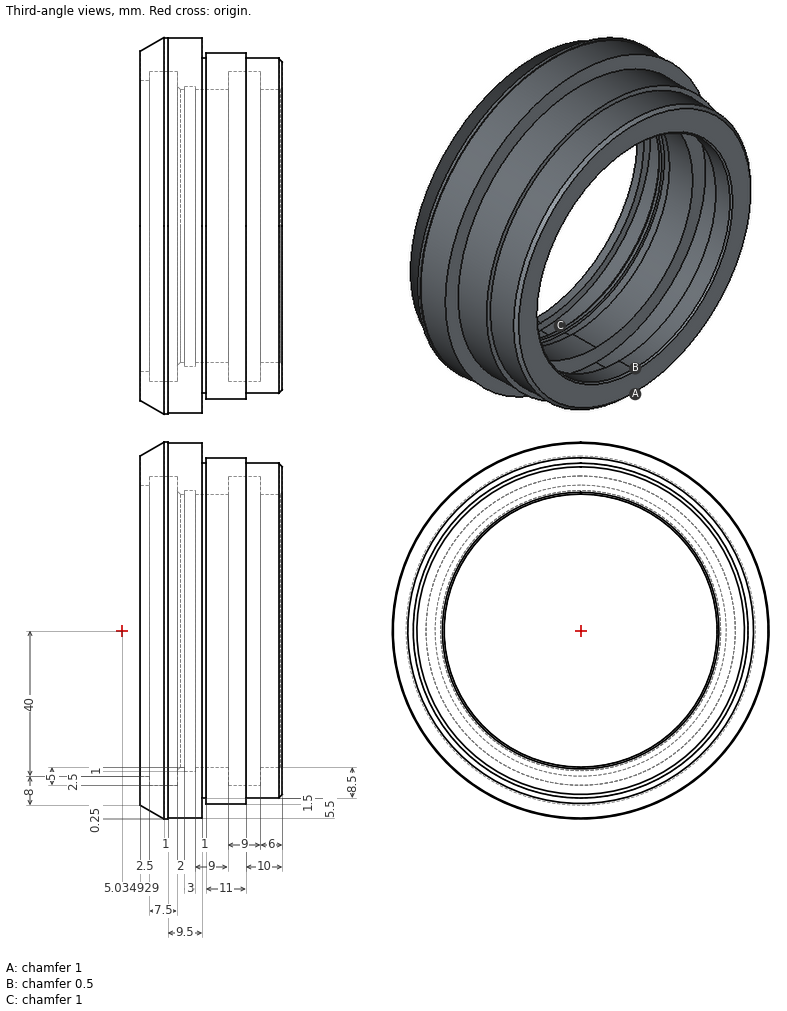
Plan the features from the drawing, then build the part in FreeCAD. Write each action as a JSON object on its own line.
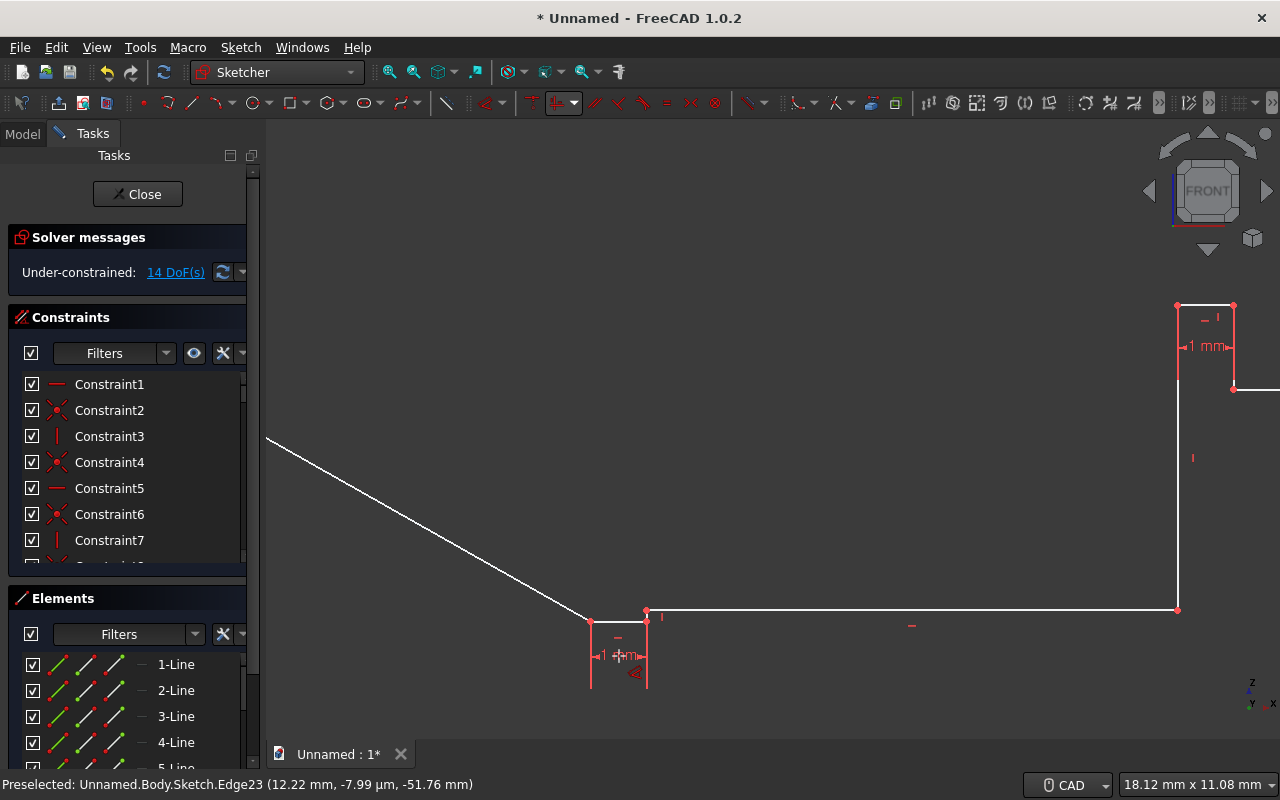
{"action": "scroll", "coordinate": [630, 626], "scroll_direction": "down", "scroll_amount": 10}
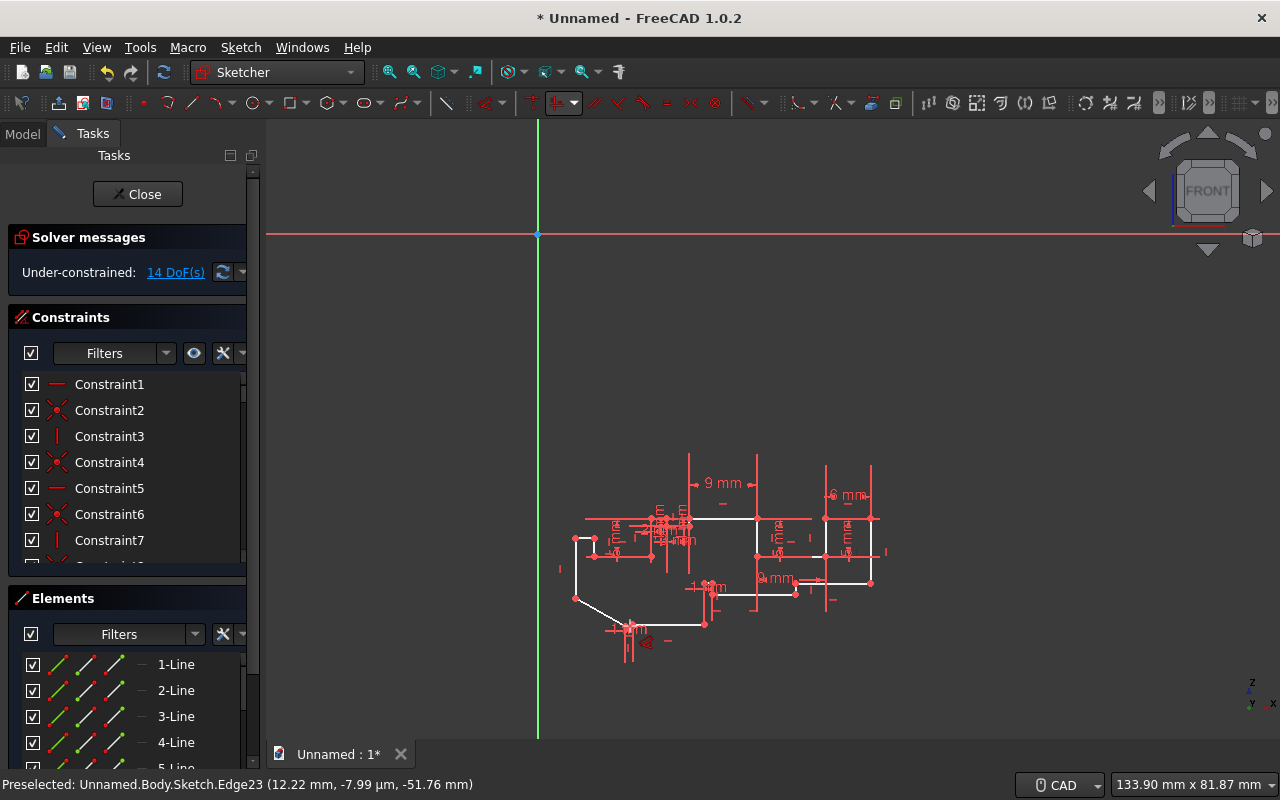
{"action": "left_click", "coordinate": [576, 580]}
{"action": "left_click", "coordinate": [610, 582]}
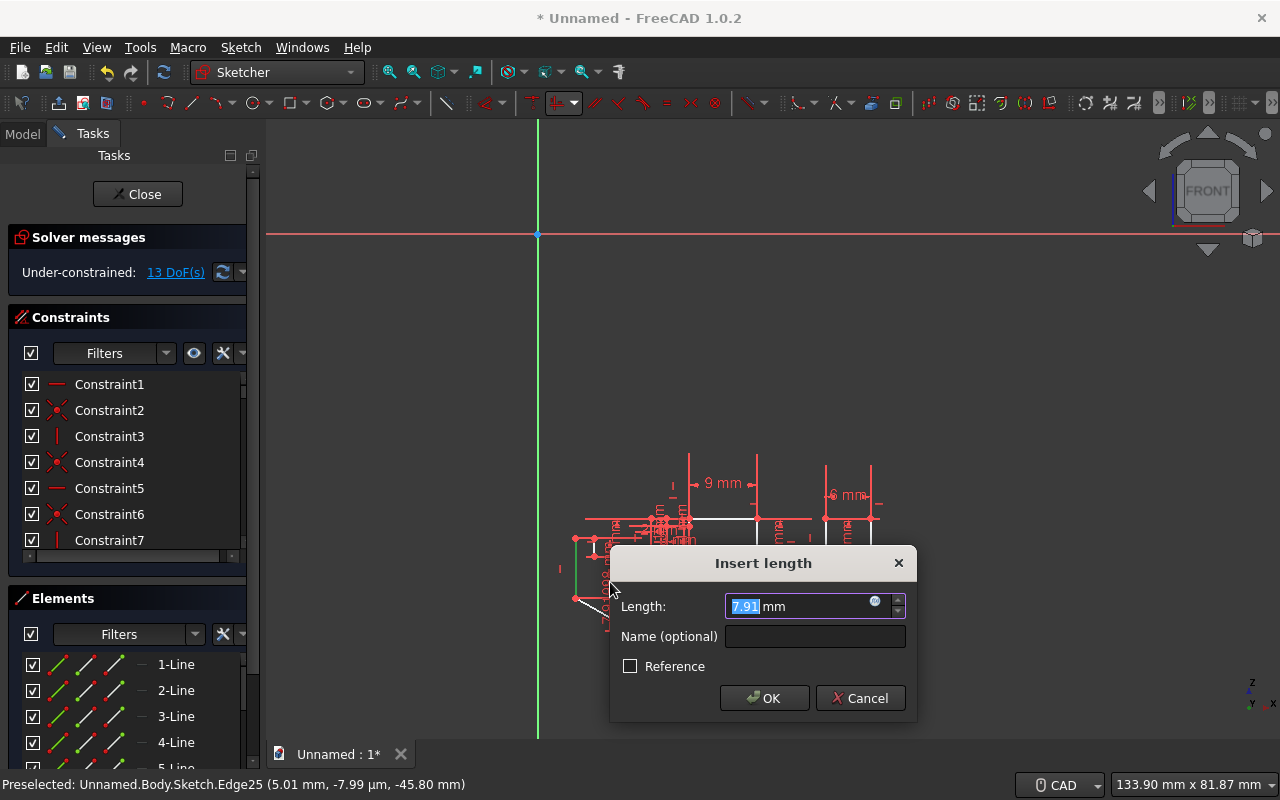
{"action": "type", "text": "8"}
{"action": "key", "text": "Return"}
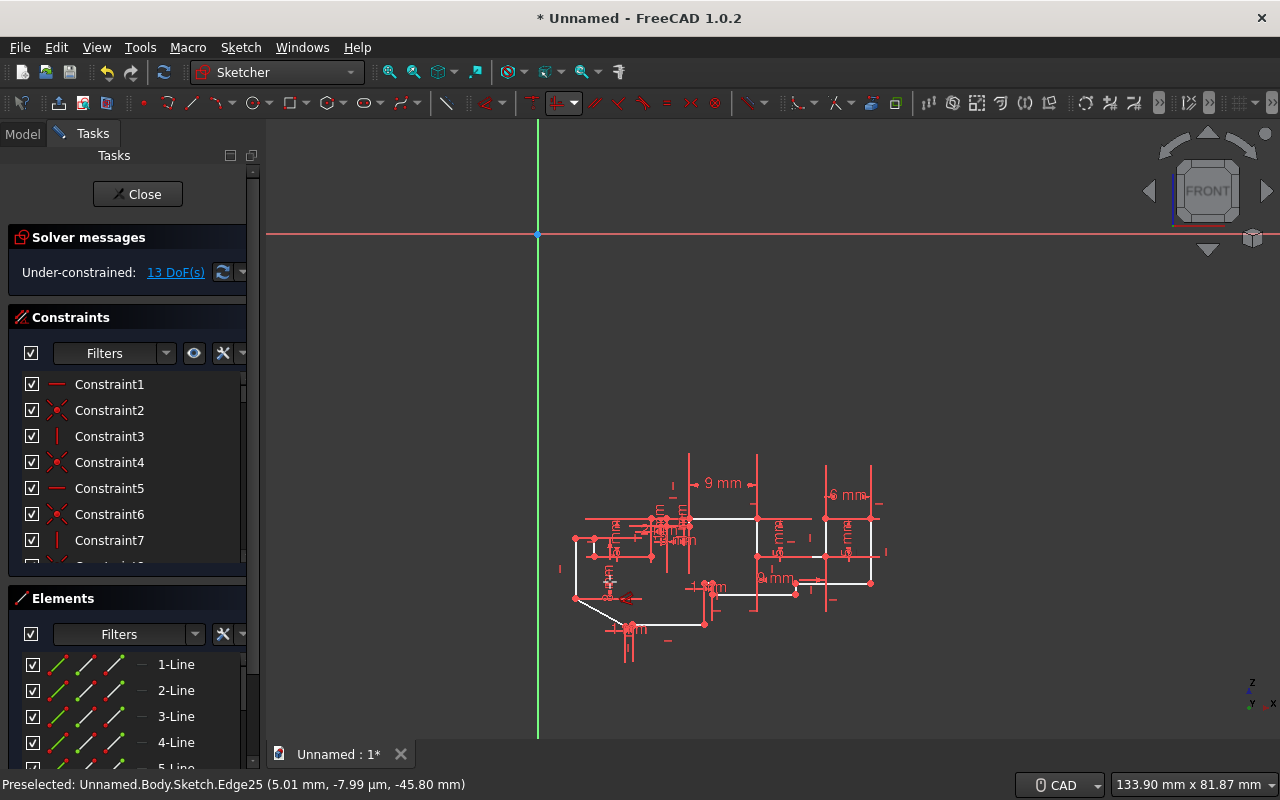
{"action": "left_click", "coordinate": [848, 584]}
{"action": "left_click", "coordinate": [833, 618]}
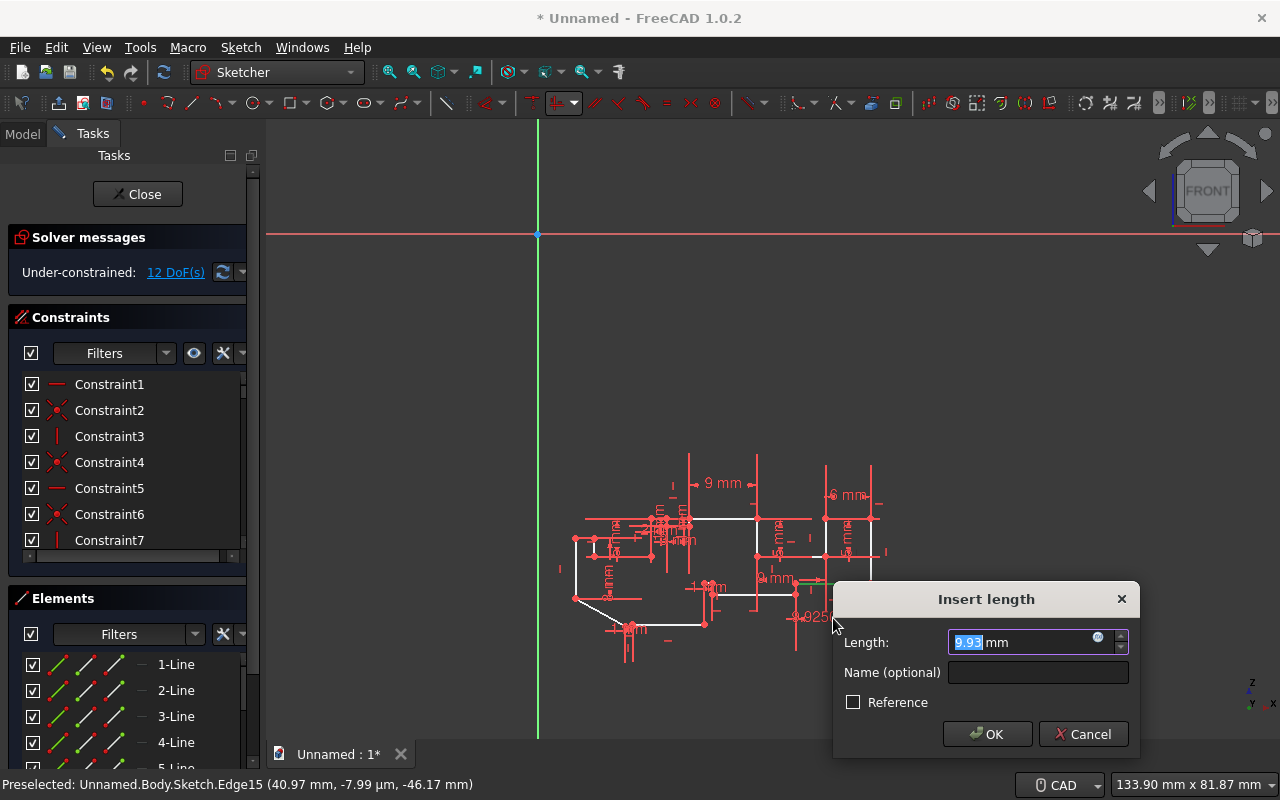
{"action": "type", "text": "10"}
{"action": "key", "text": "Return"}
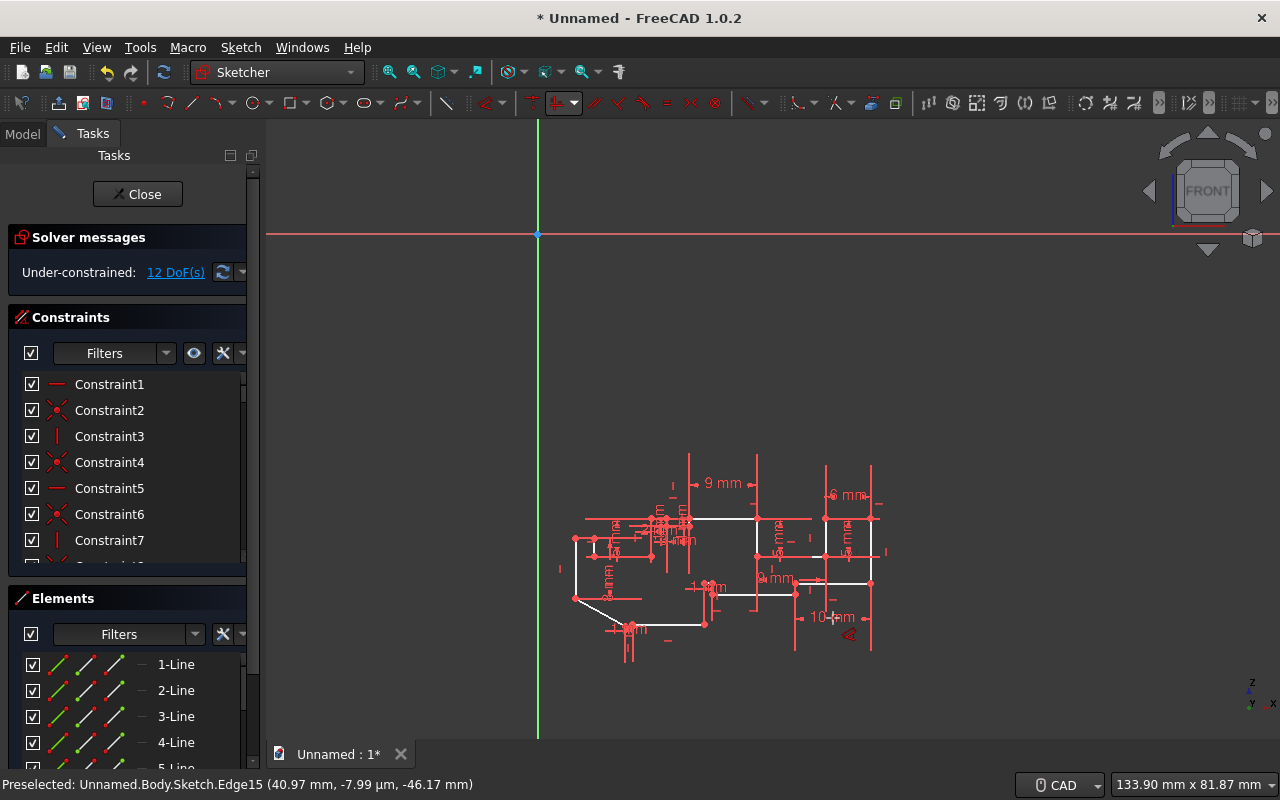
{"action": "left_click", "coordinate": [770, 595]}
{"action": "left_click", "coordinate": [754, 629]}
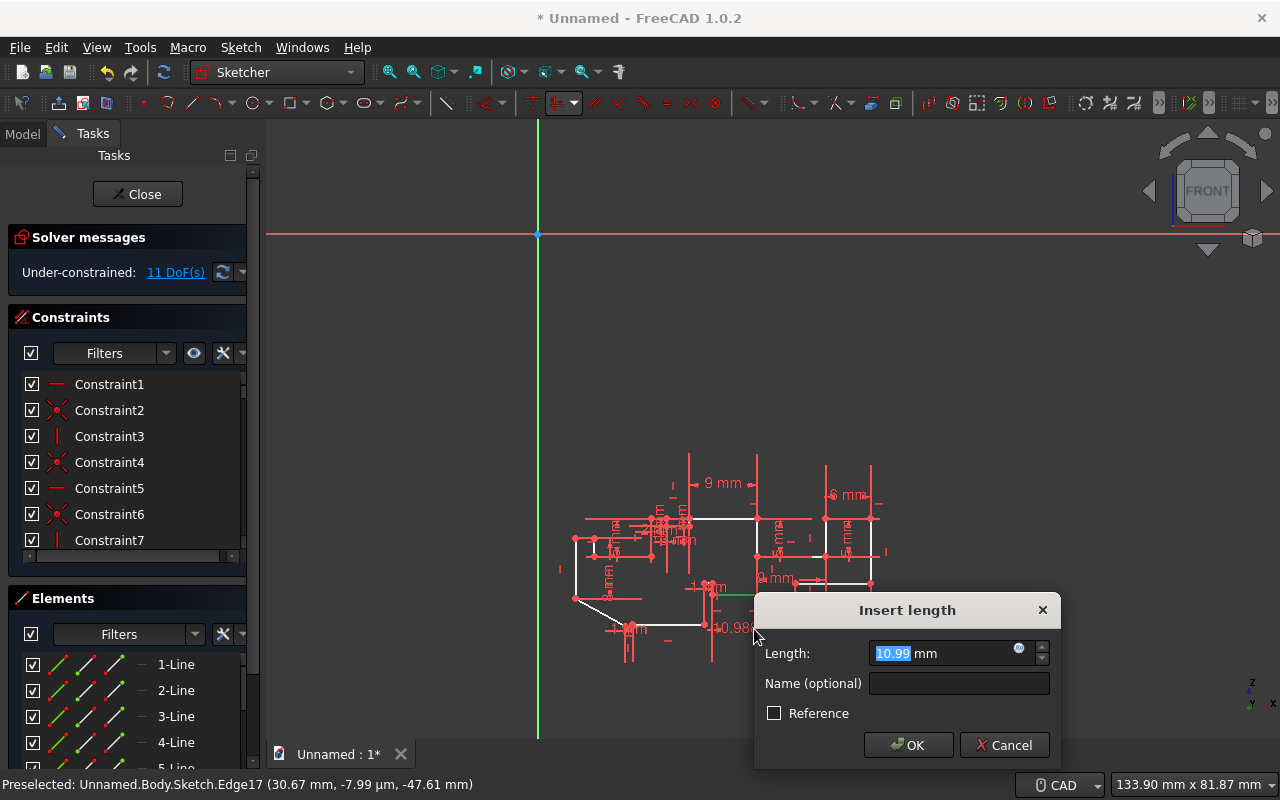
{"action": "type", "text": "11"}
{"action": "key", "text": "Return"}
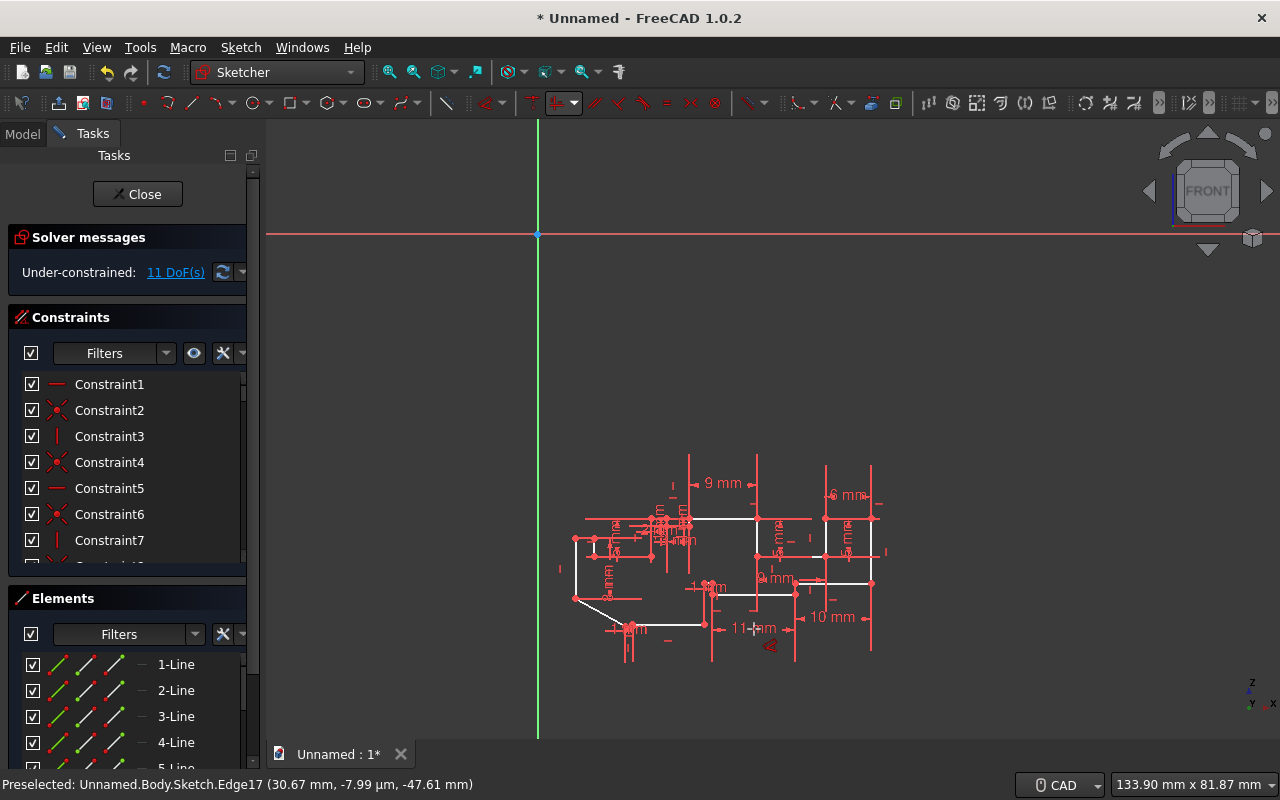
{"action": "scroll", "coordinate": [585, 538], "scroll_direction": "up", "scroll_amount": 4}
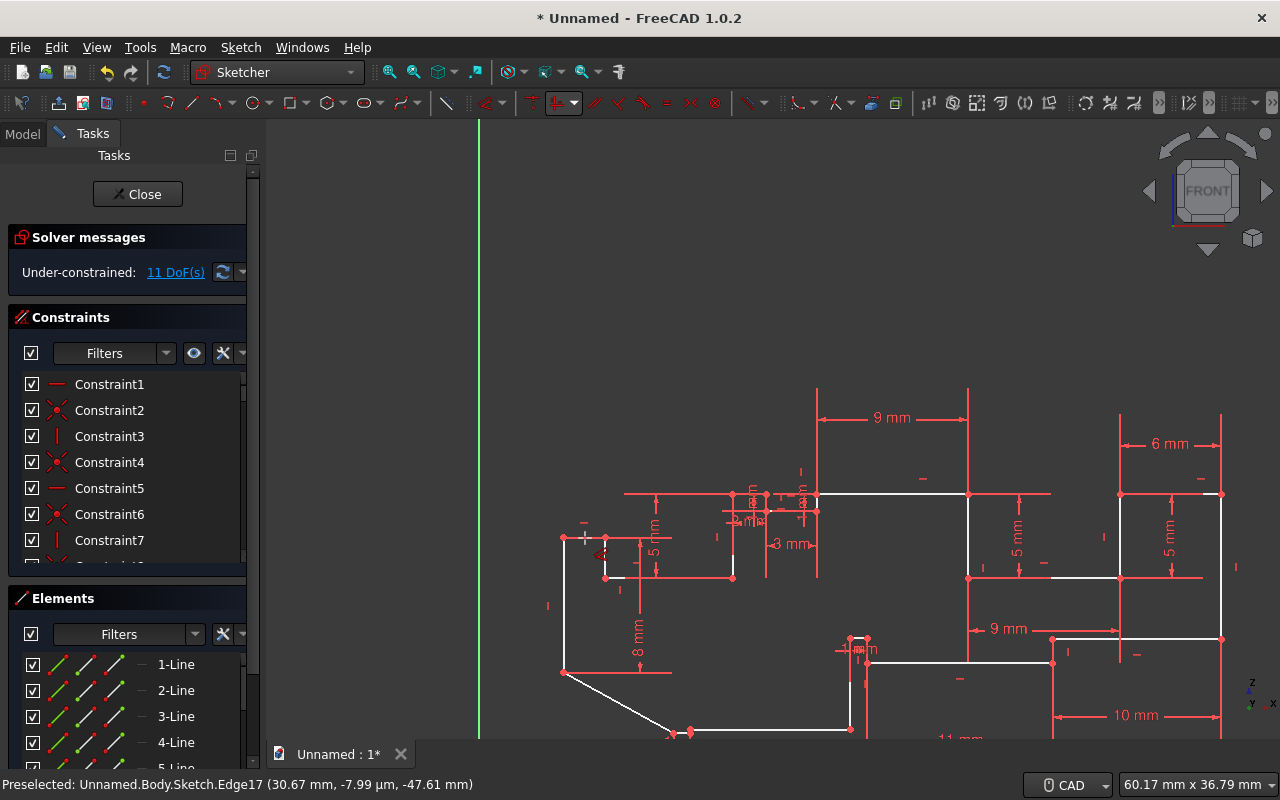
{"action": "left_click", "coordinate": [585, 538]}
{"action": "left_click", "coordinate": [585, 572]}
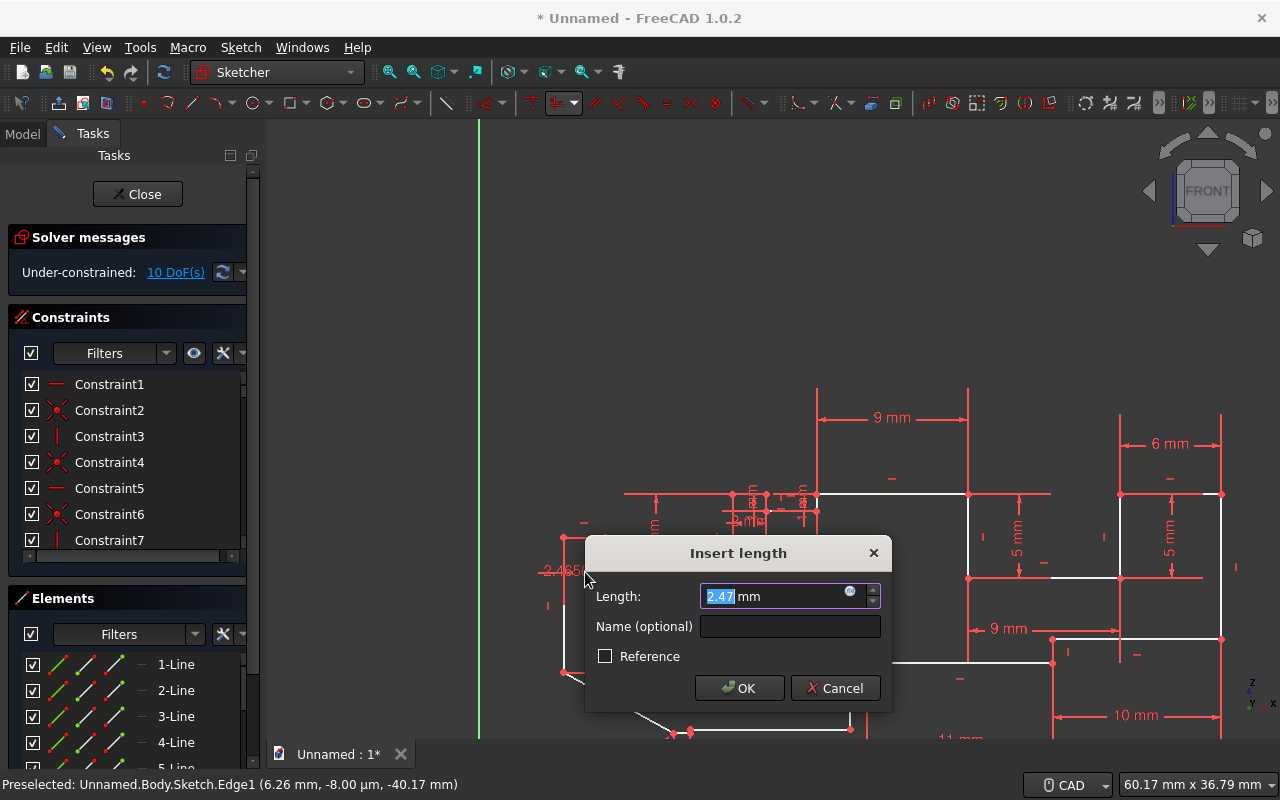
{"action": "type", "text": "2.5"}
{"action": "key", "text": "Return"}